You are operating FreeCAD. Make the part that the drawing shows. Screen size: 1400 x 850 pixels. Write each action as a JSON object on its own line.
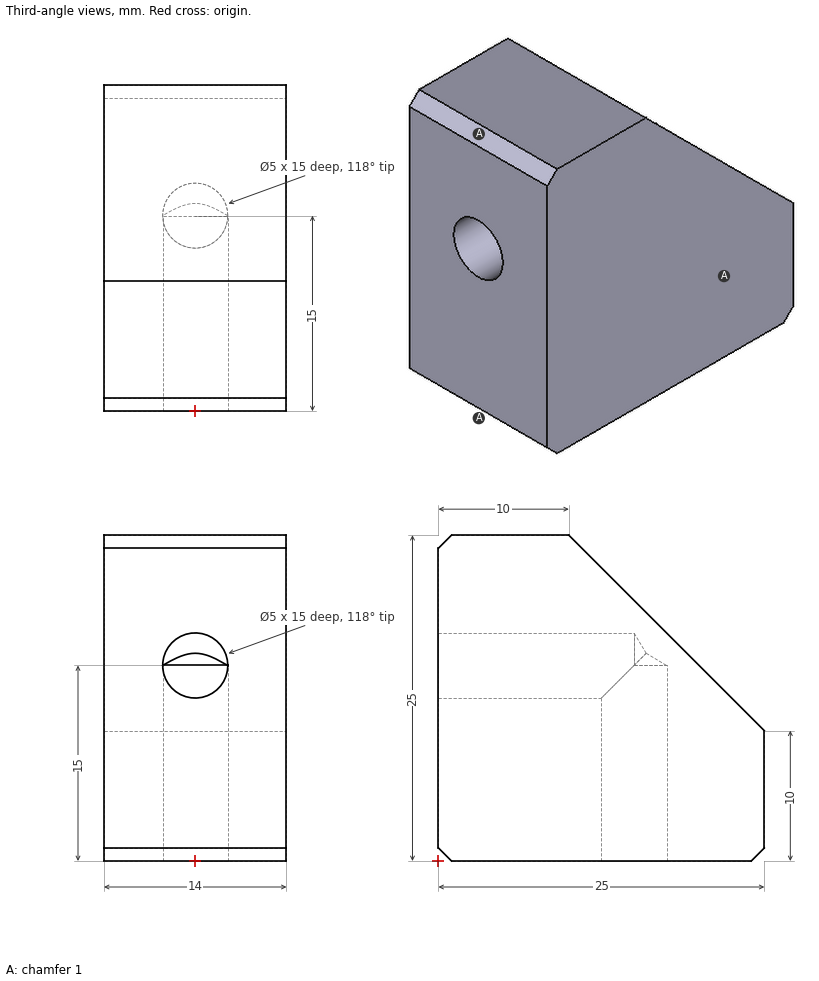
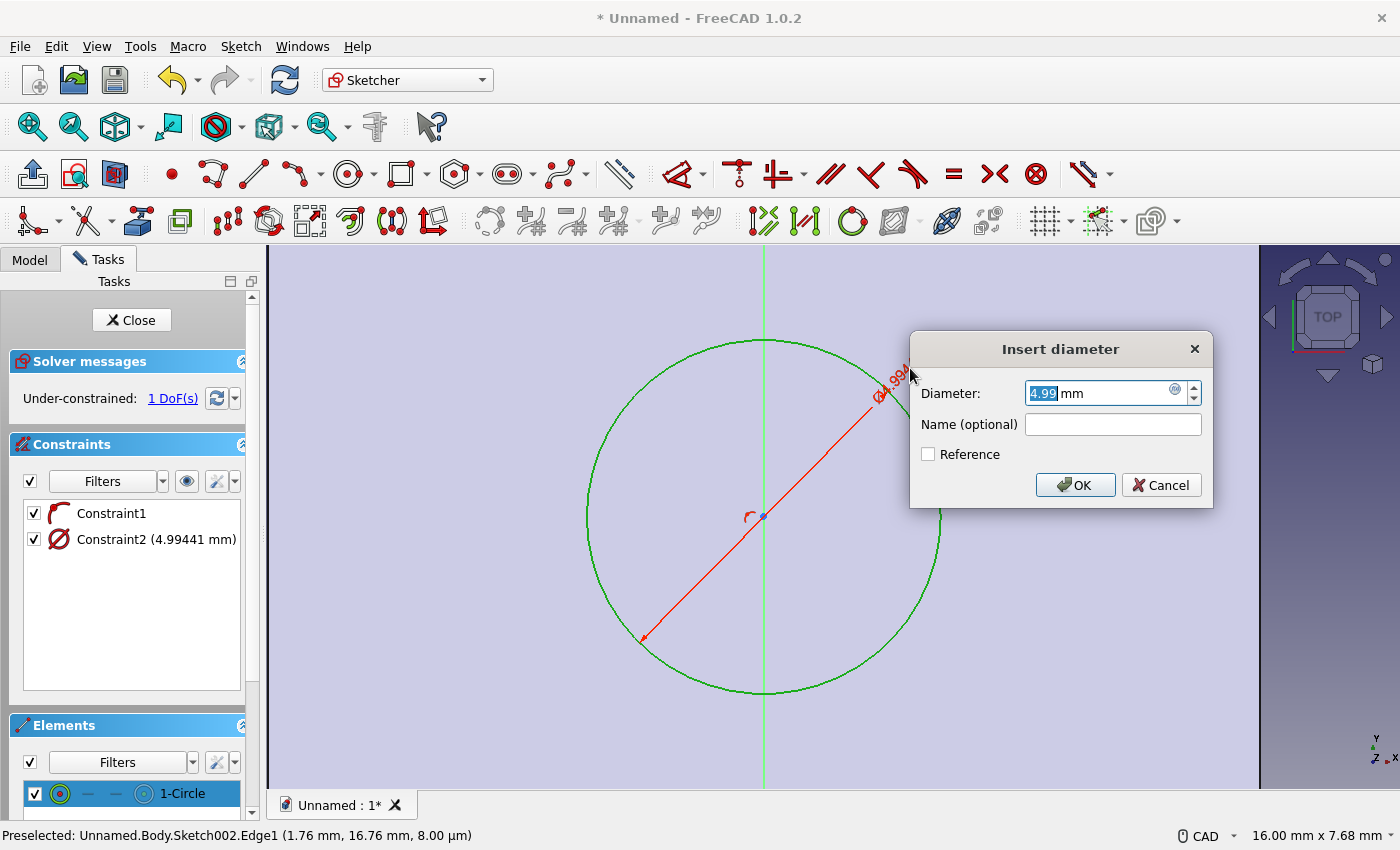
{"action": "type", "text": "5"}
{"action": "key", "text": "Return"}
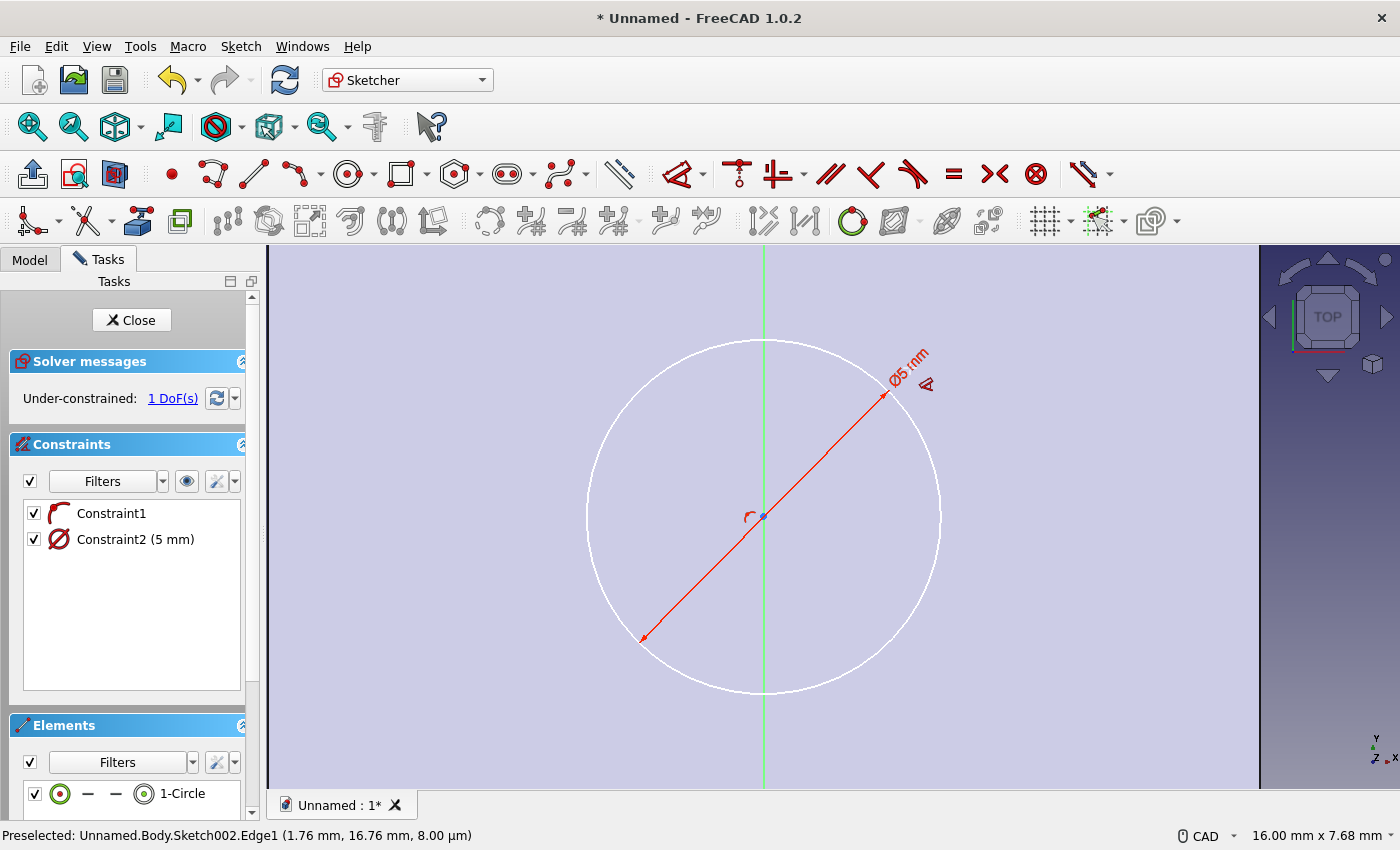
{"action": "left_click", "coordinate": [764, 517]}
{"action": "left_click", "coordinate": [798, 639]}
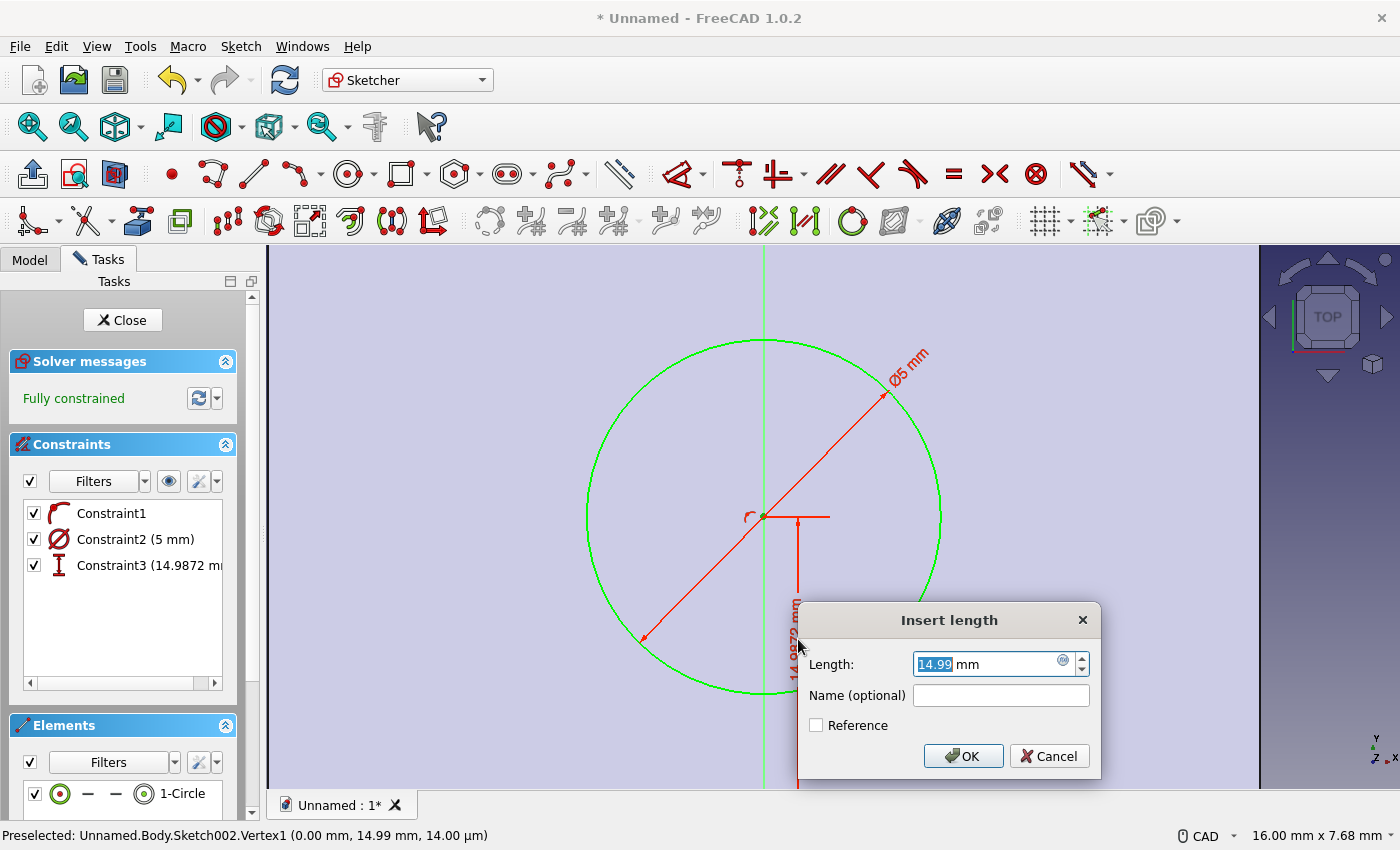
{"action": "type", "text": "15"}
{"action": "key", "text": "Return"}
{"action": "key", "text": "Escape"}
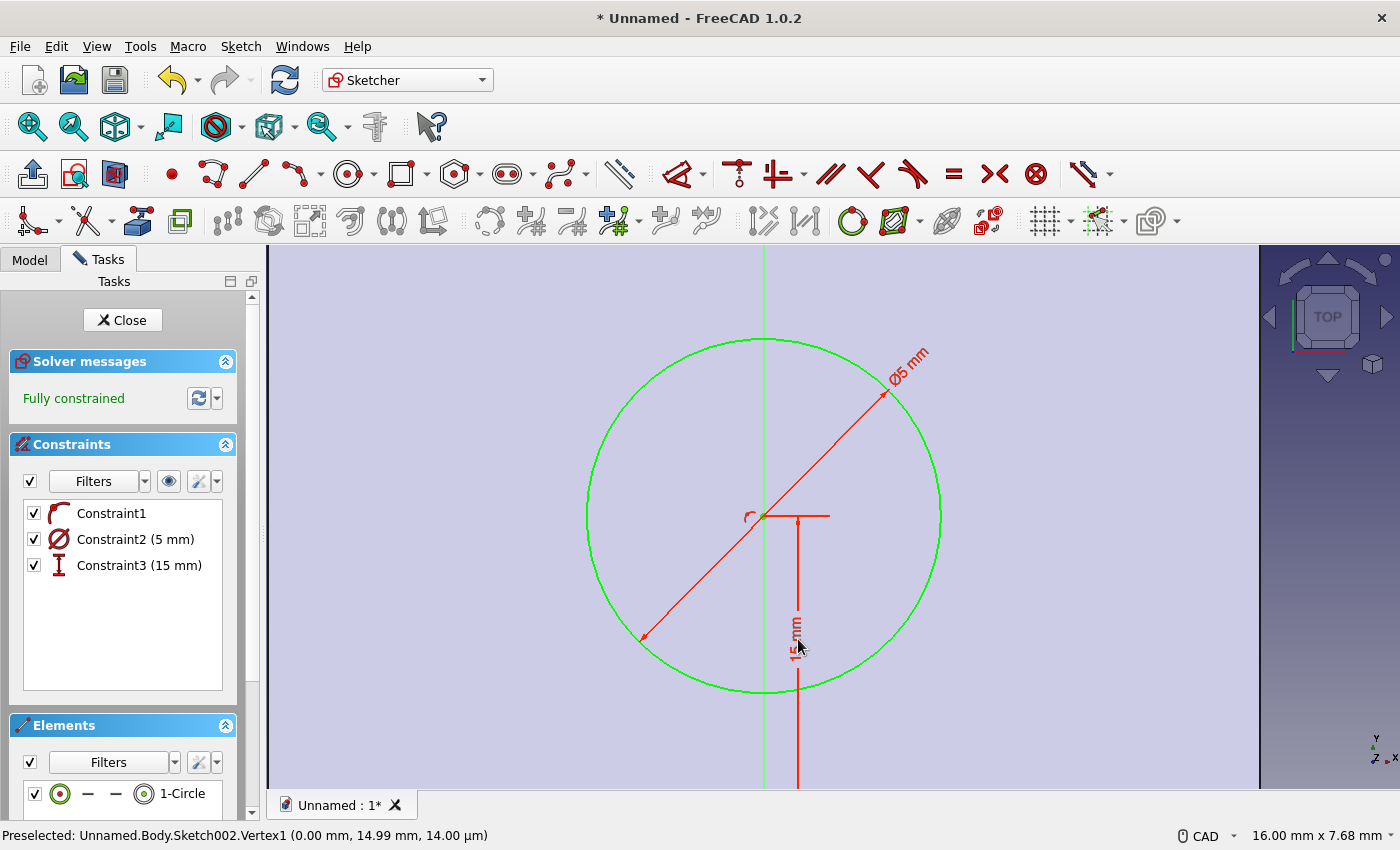
{"action": "left_click", "coordinate": [123, 320]}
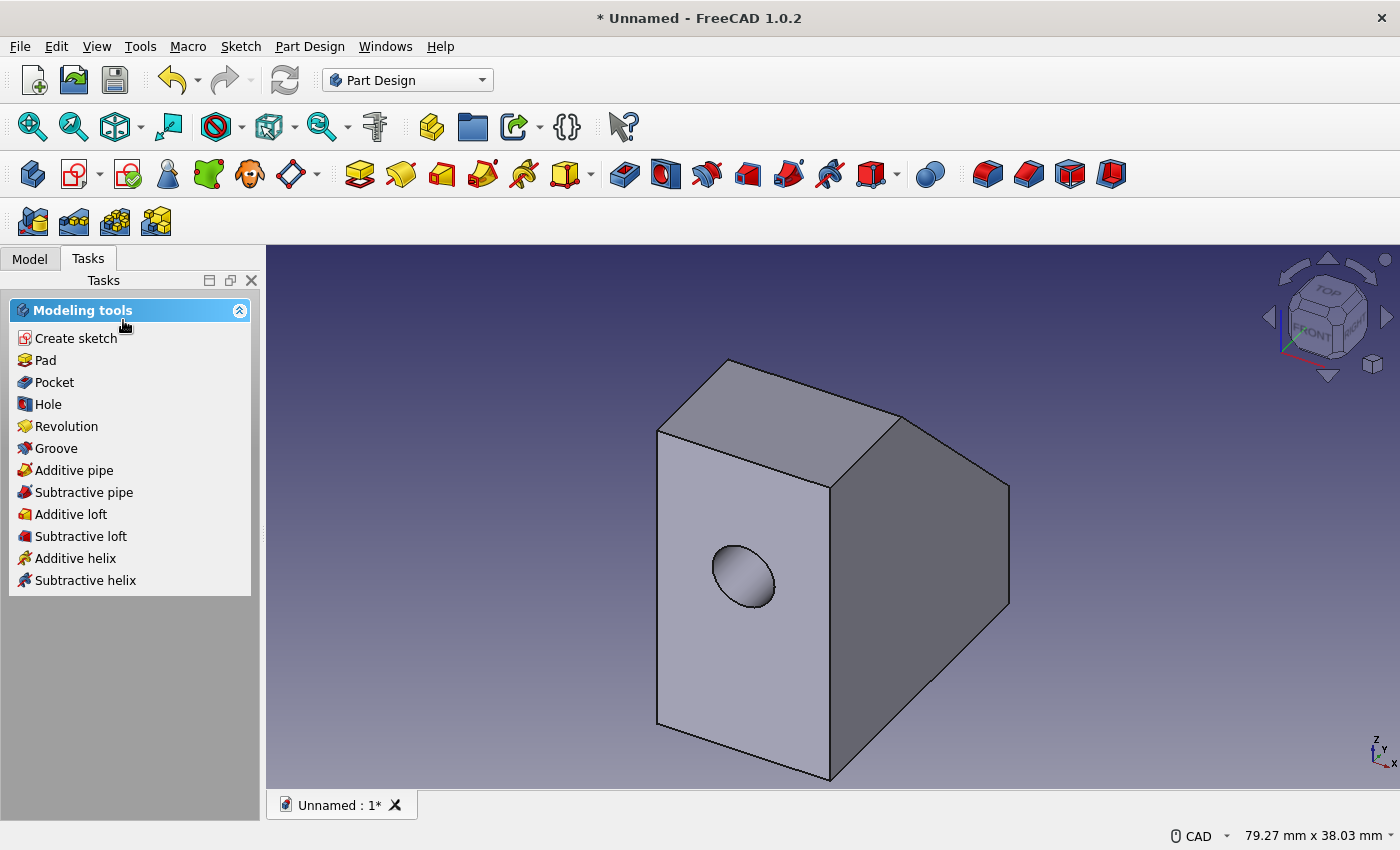
{"action": "left_click", "coordinate": [666, 174]}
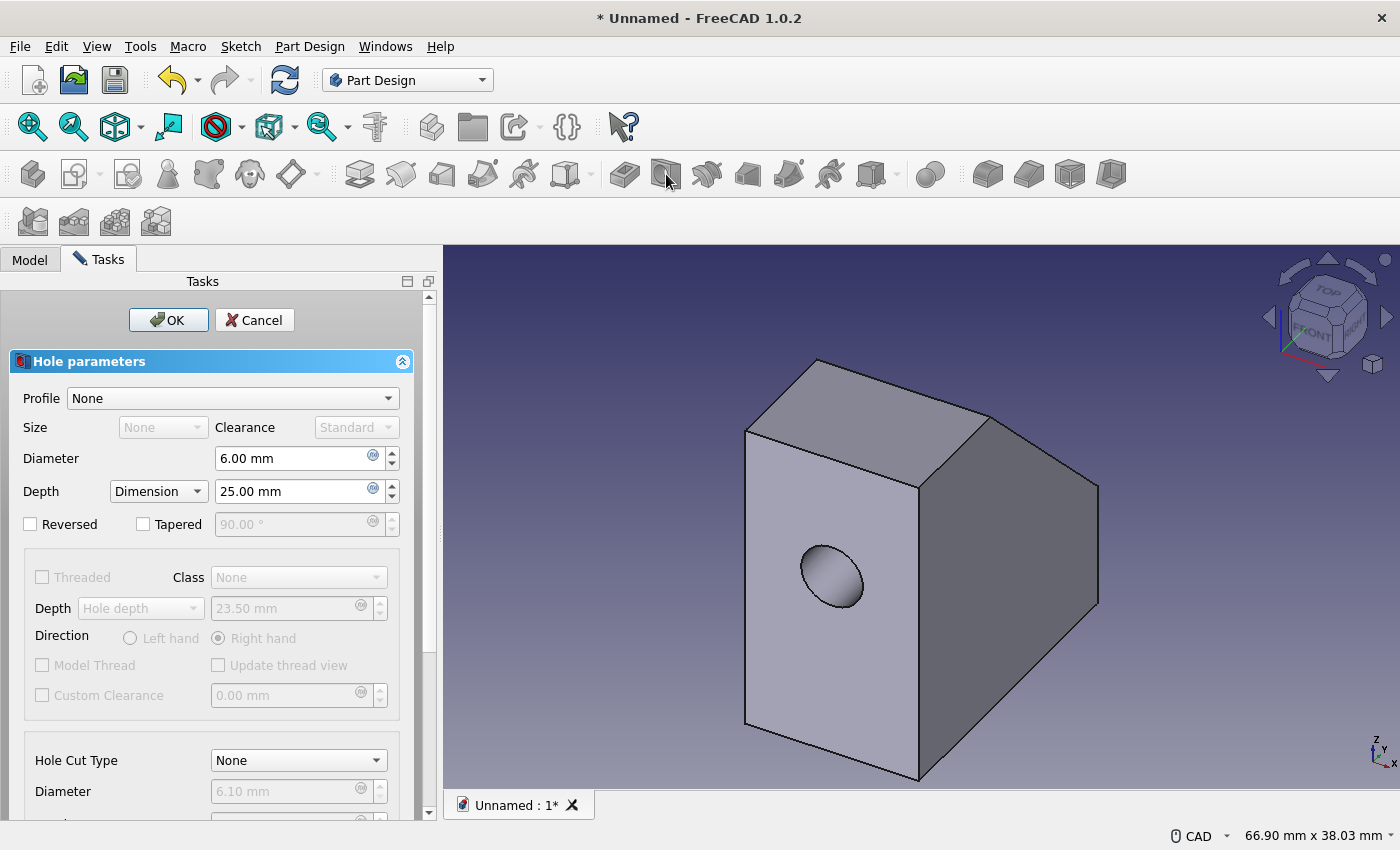
{"action": "triple_click", "coordinate": [300, 458]}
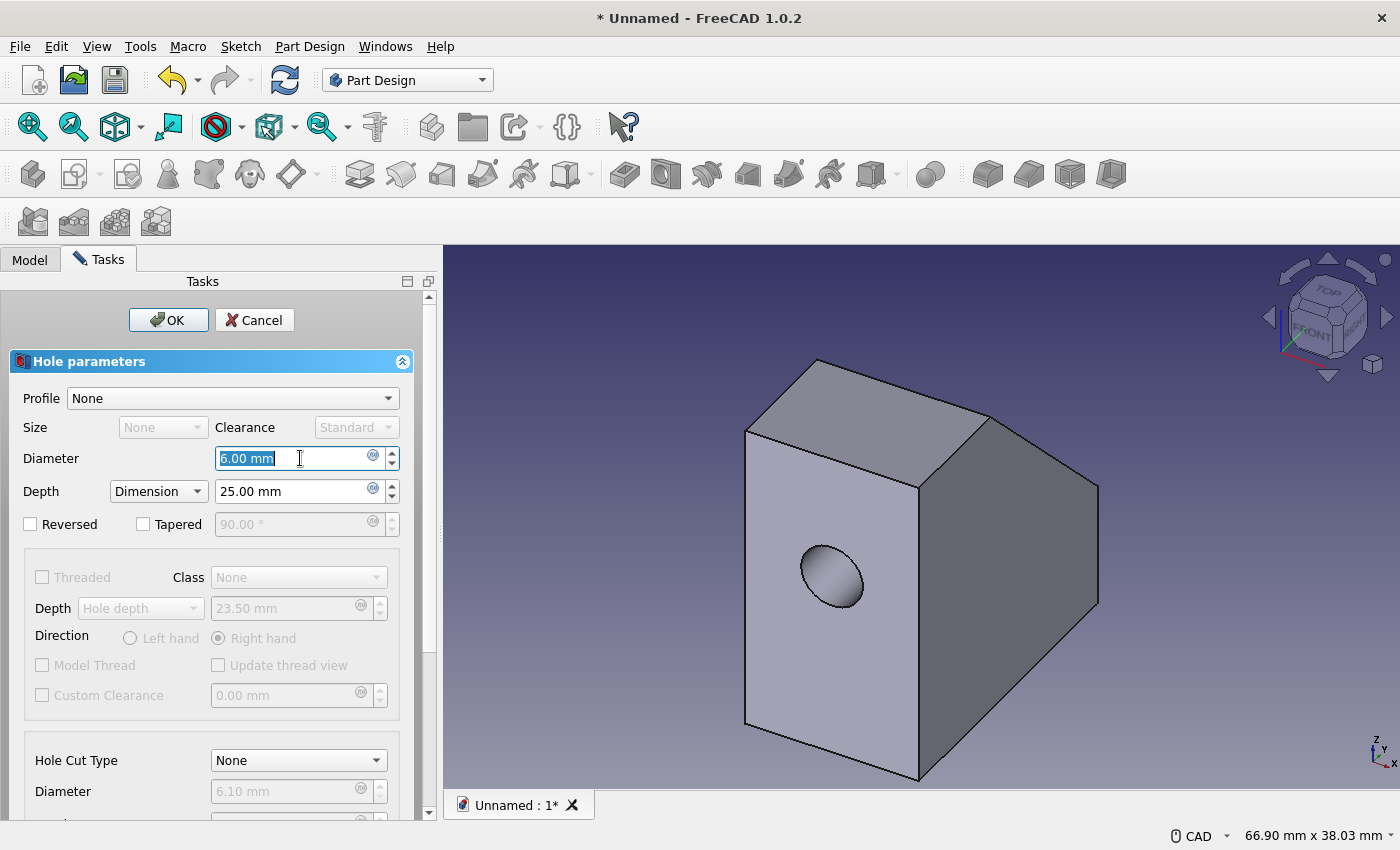
{"action": "type", "text": "5"}
{"action": "key", "text": "Tab"}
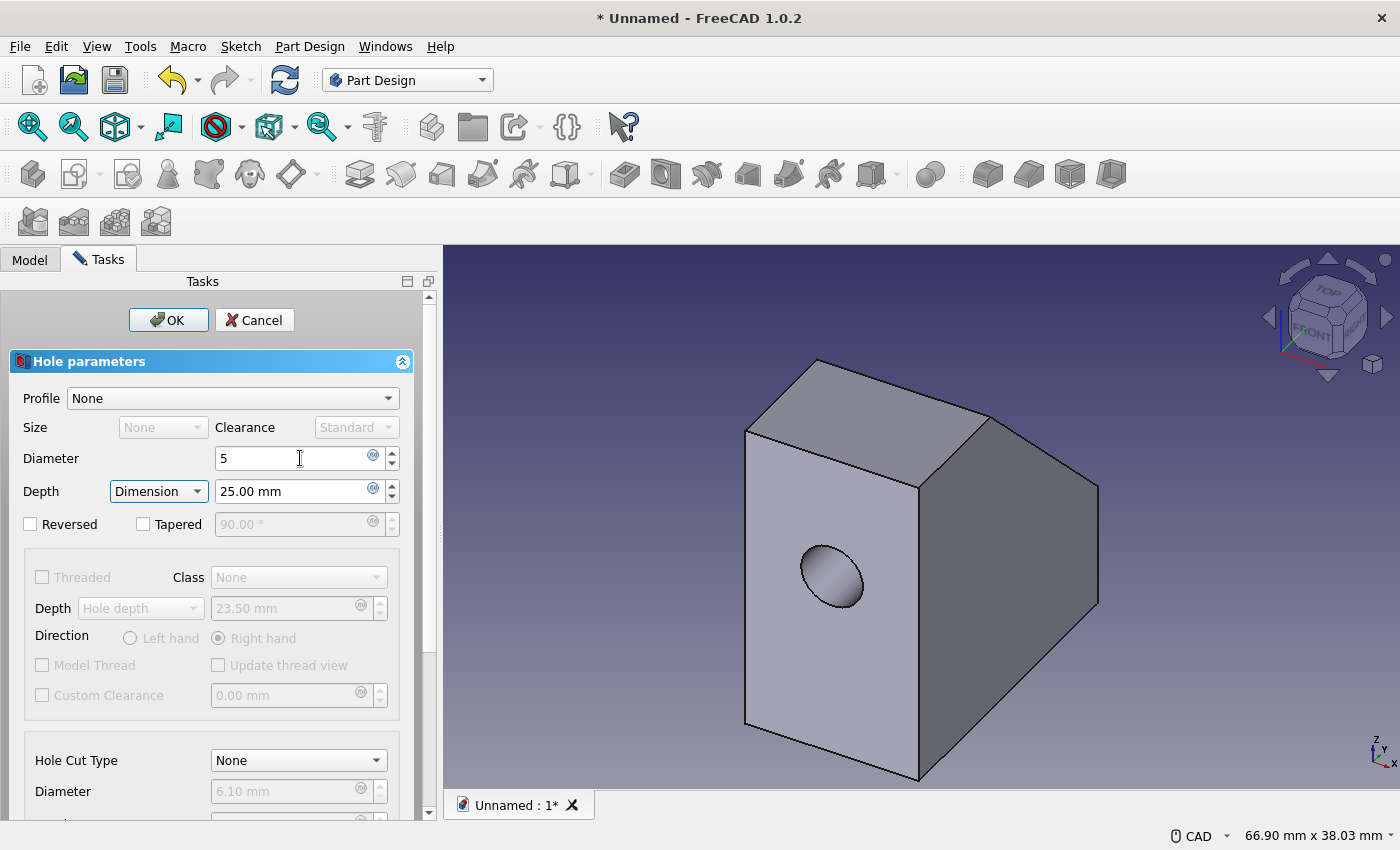
{"action": "triple_click", "coordinate": [300, 492]}